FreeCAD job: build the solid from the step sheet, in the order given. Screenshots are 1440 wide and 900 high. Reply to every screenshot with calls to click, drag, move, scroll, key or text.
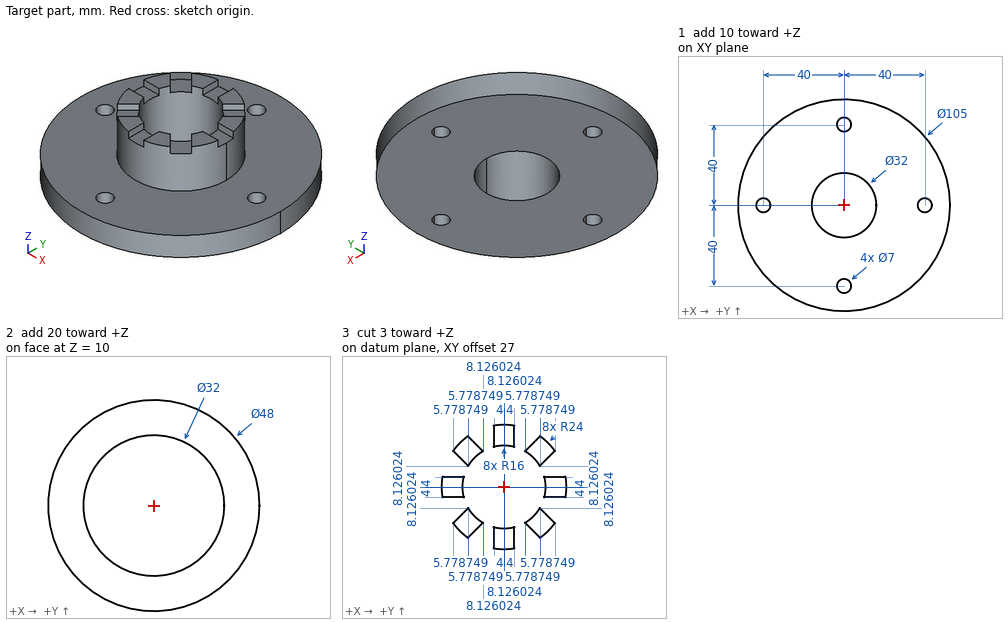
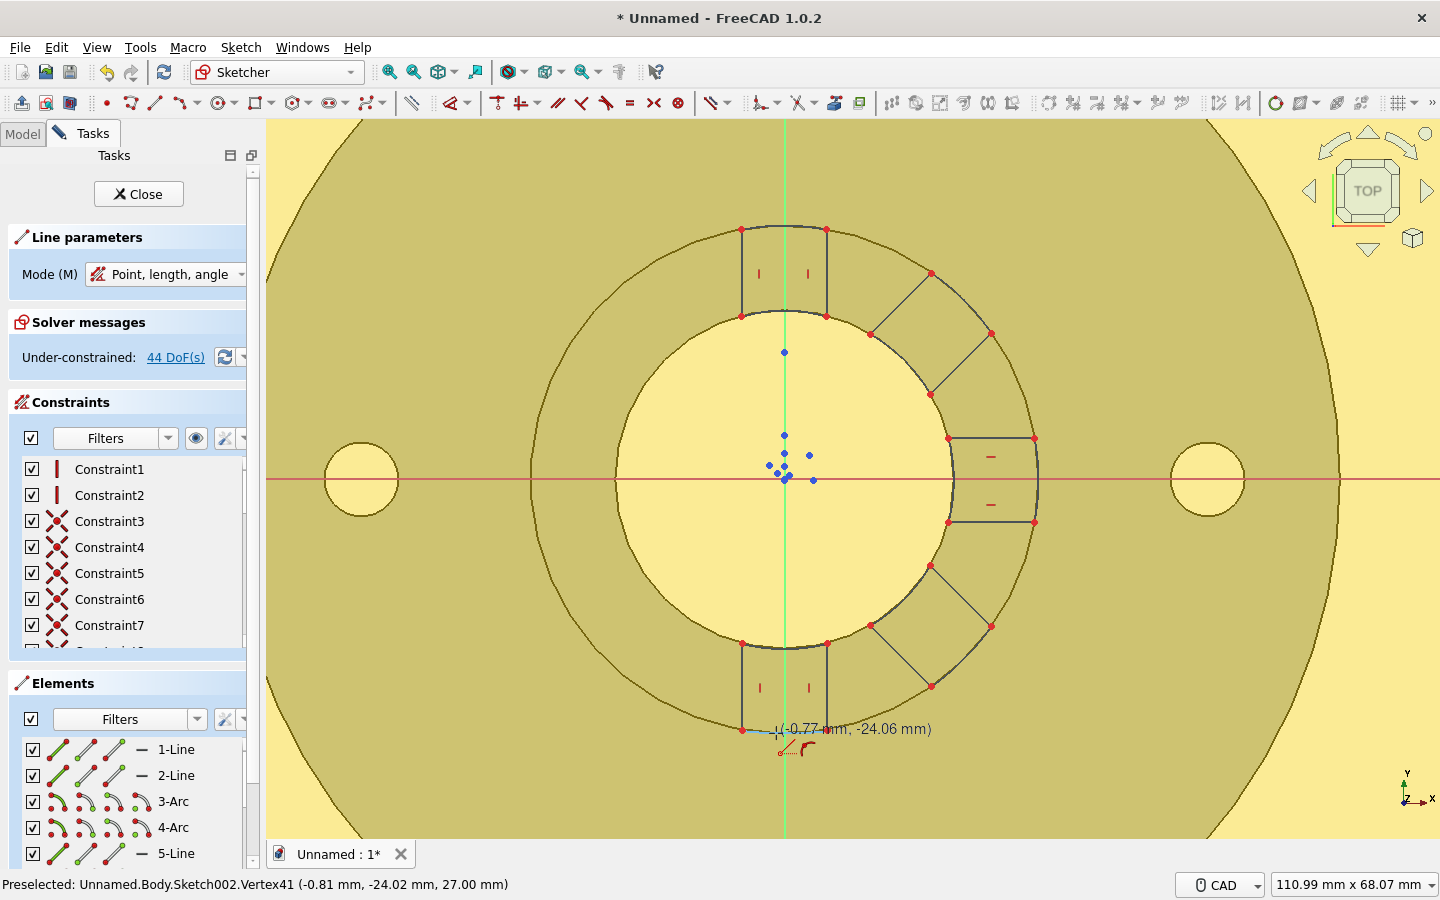
click(637, 686)
click(699, 625)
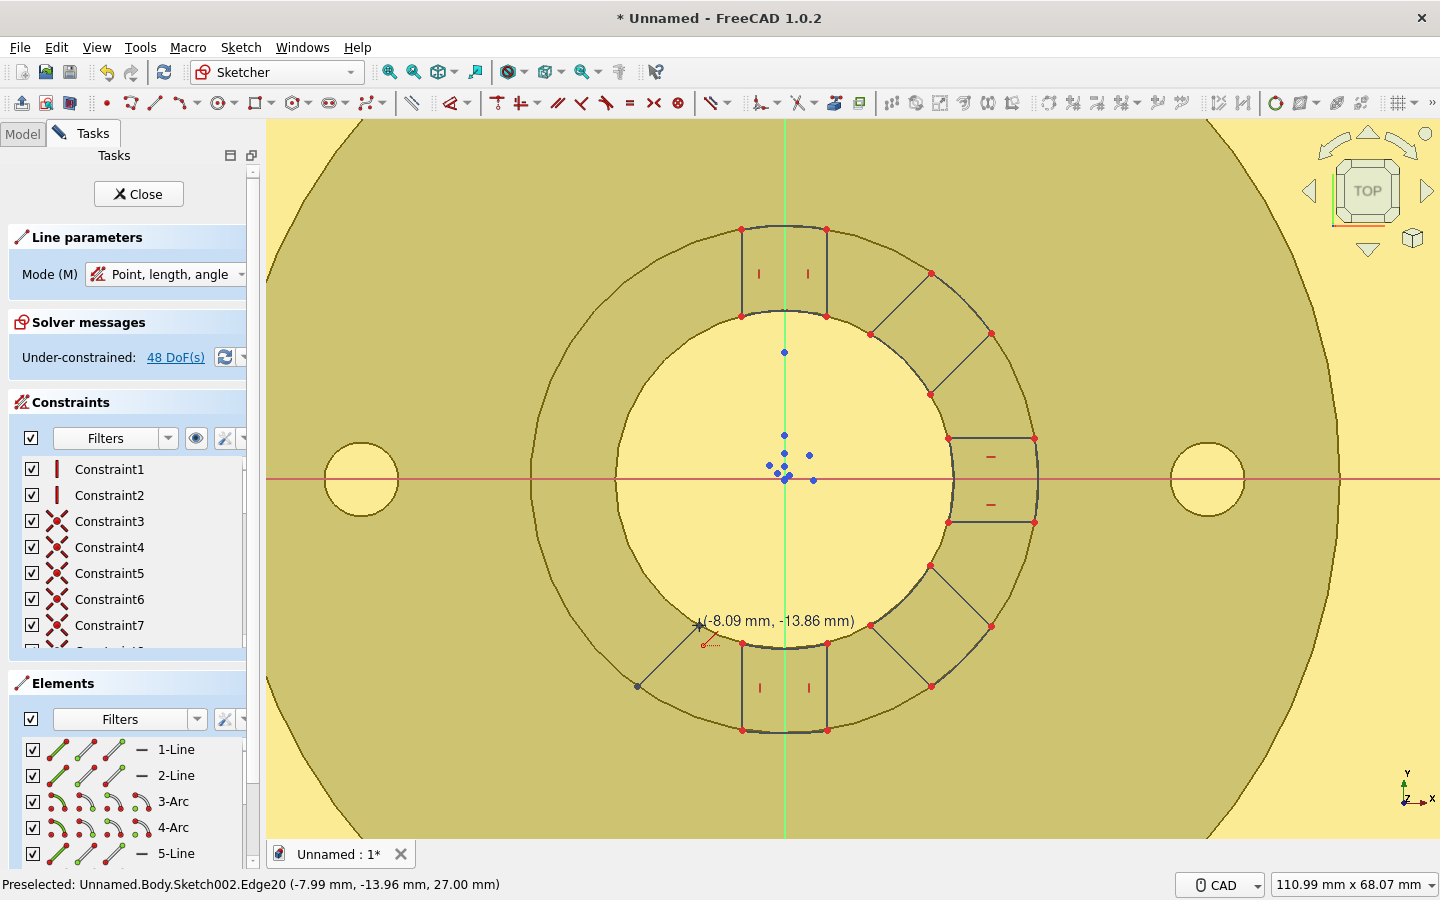
click(639, 565)
click(578, 626)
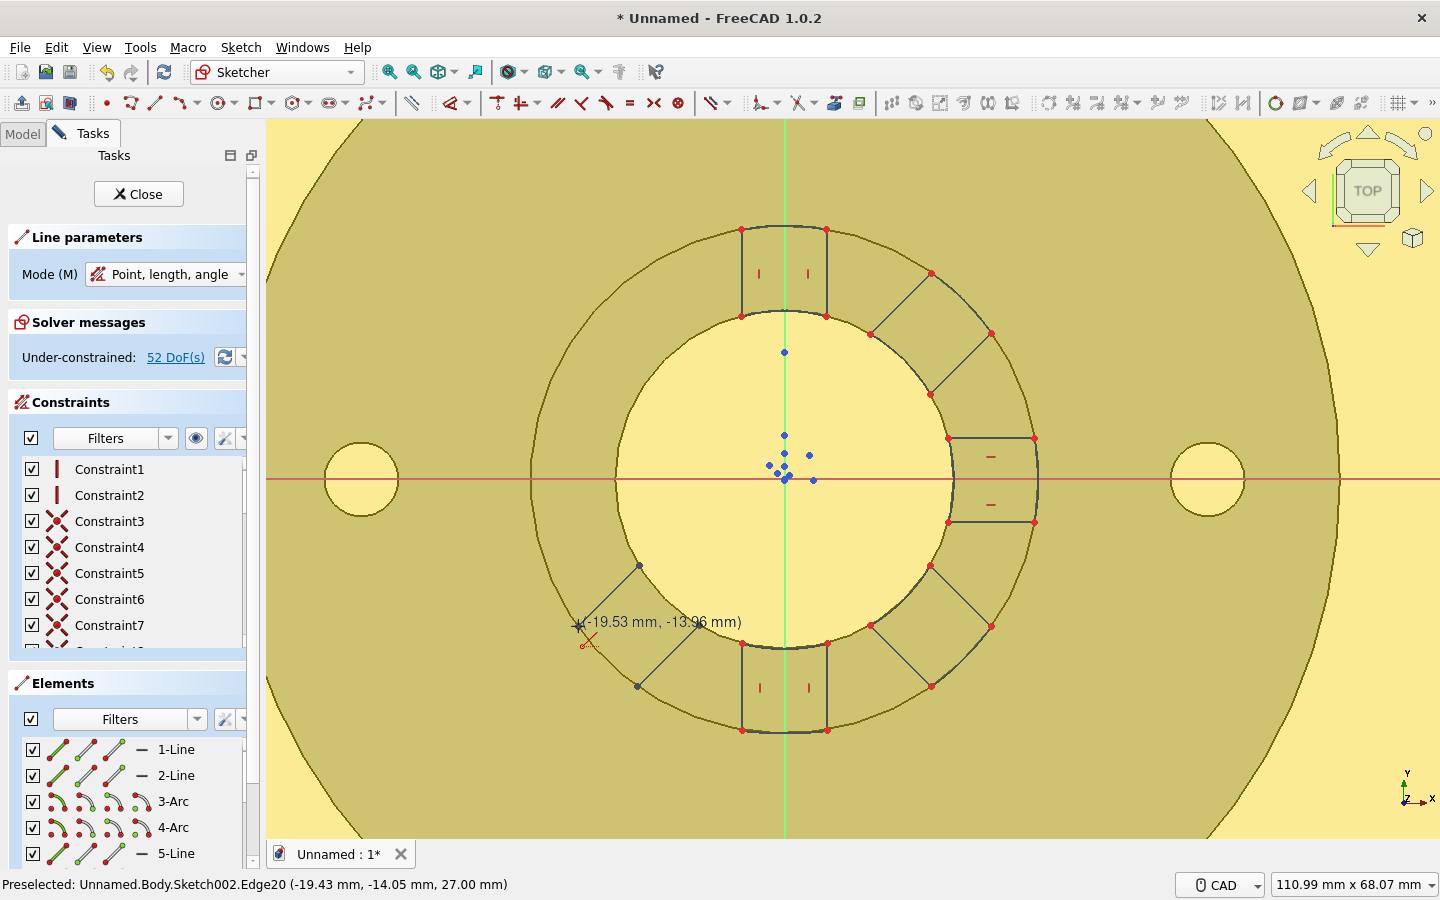
click(180, 104)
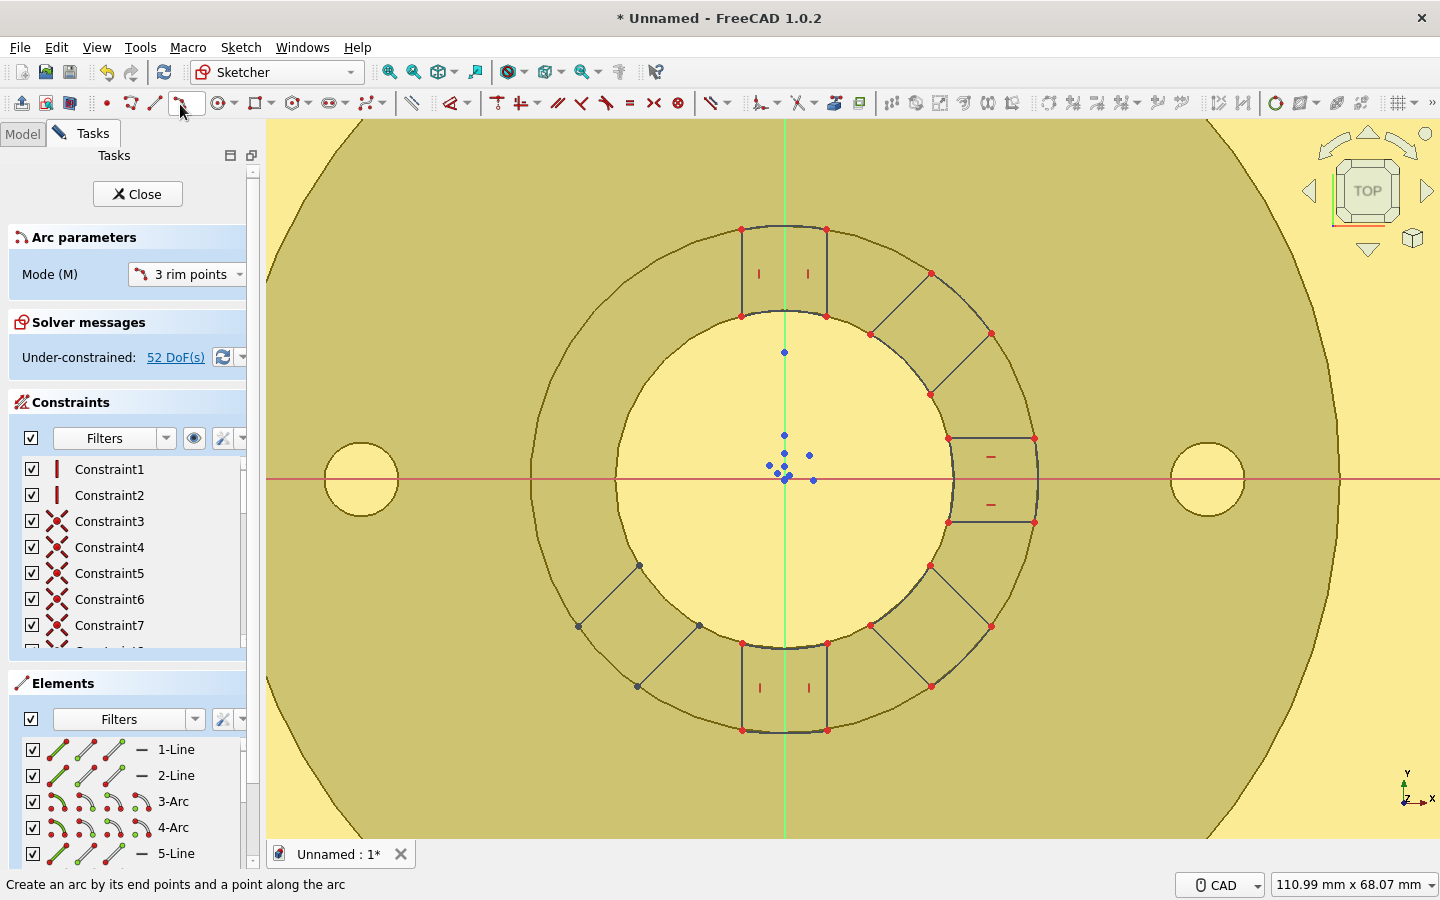
click(699, 626)
click(639, 566)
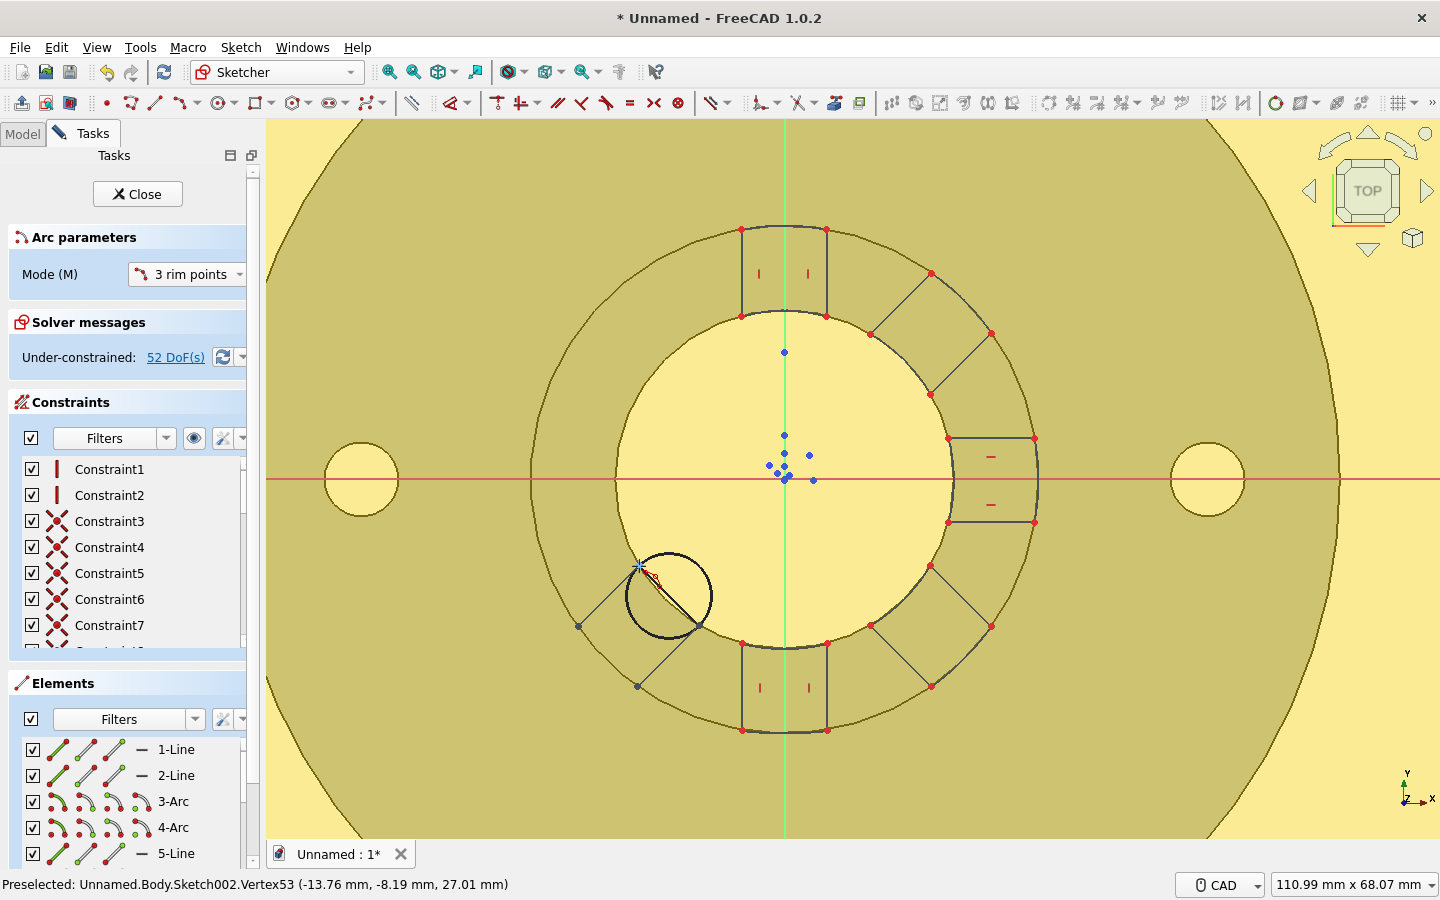
scroll(665, 599, up, 6)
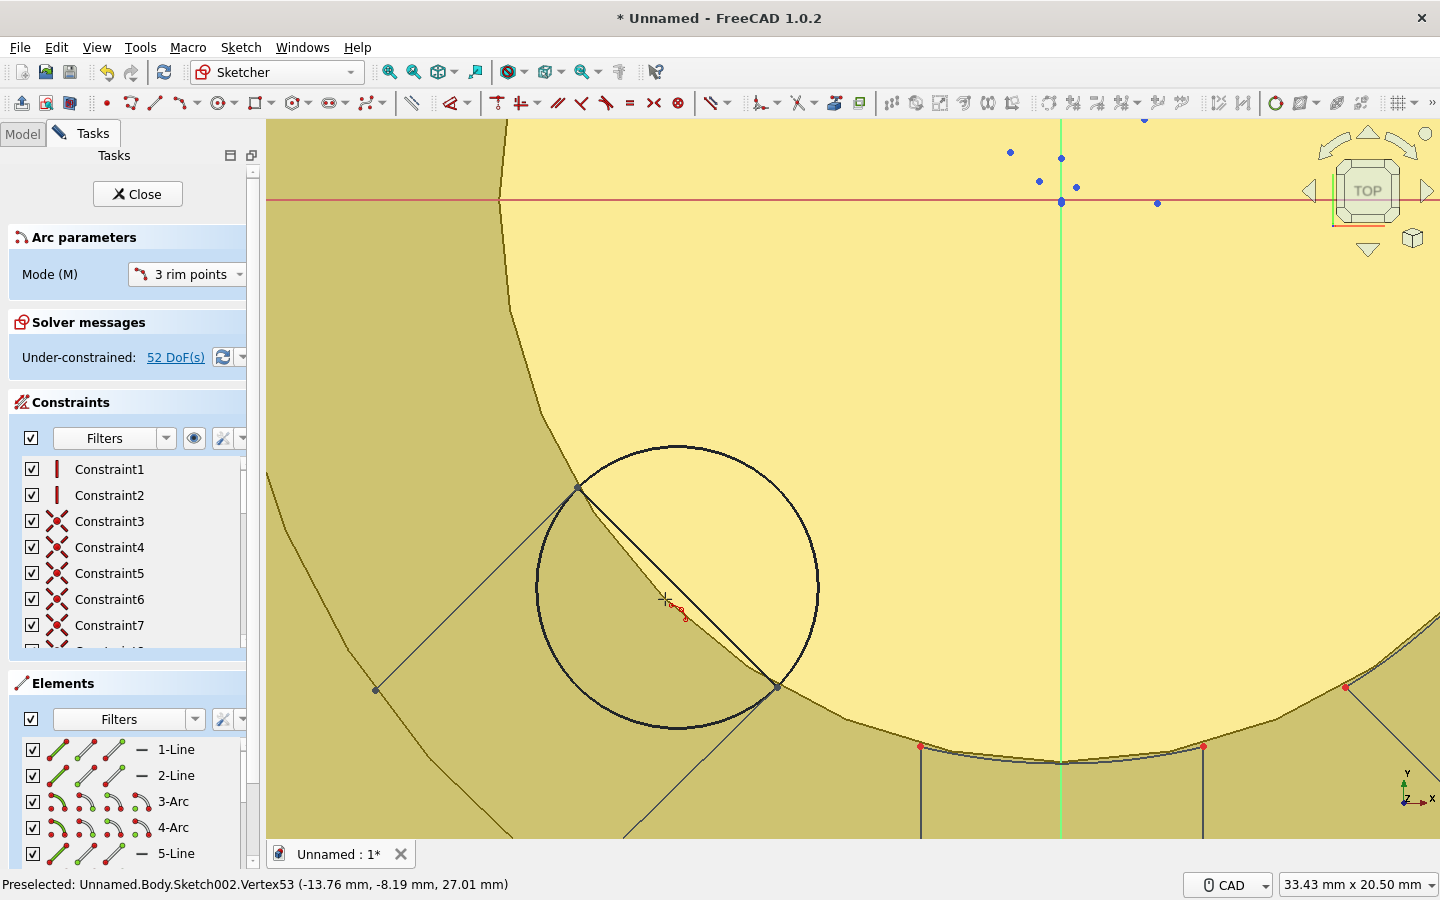
click(664, 598)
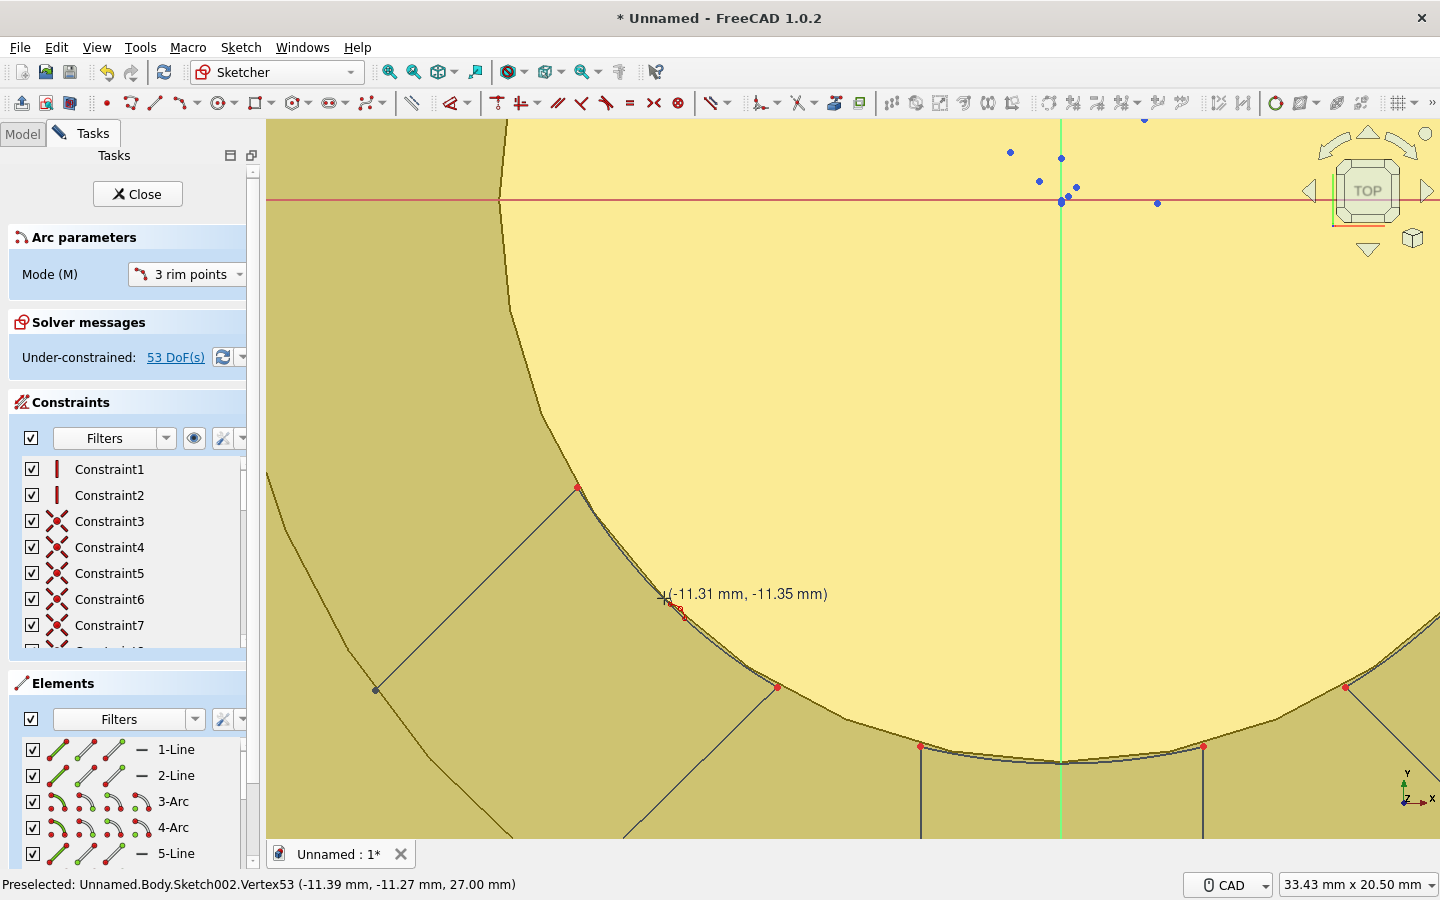
click(375, 690)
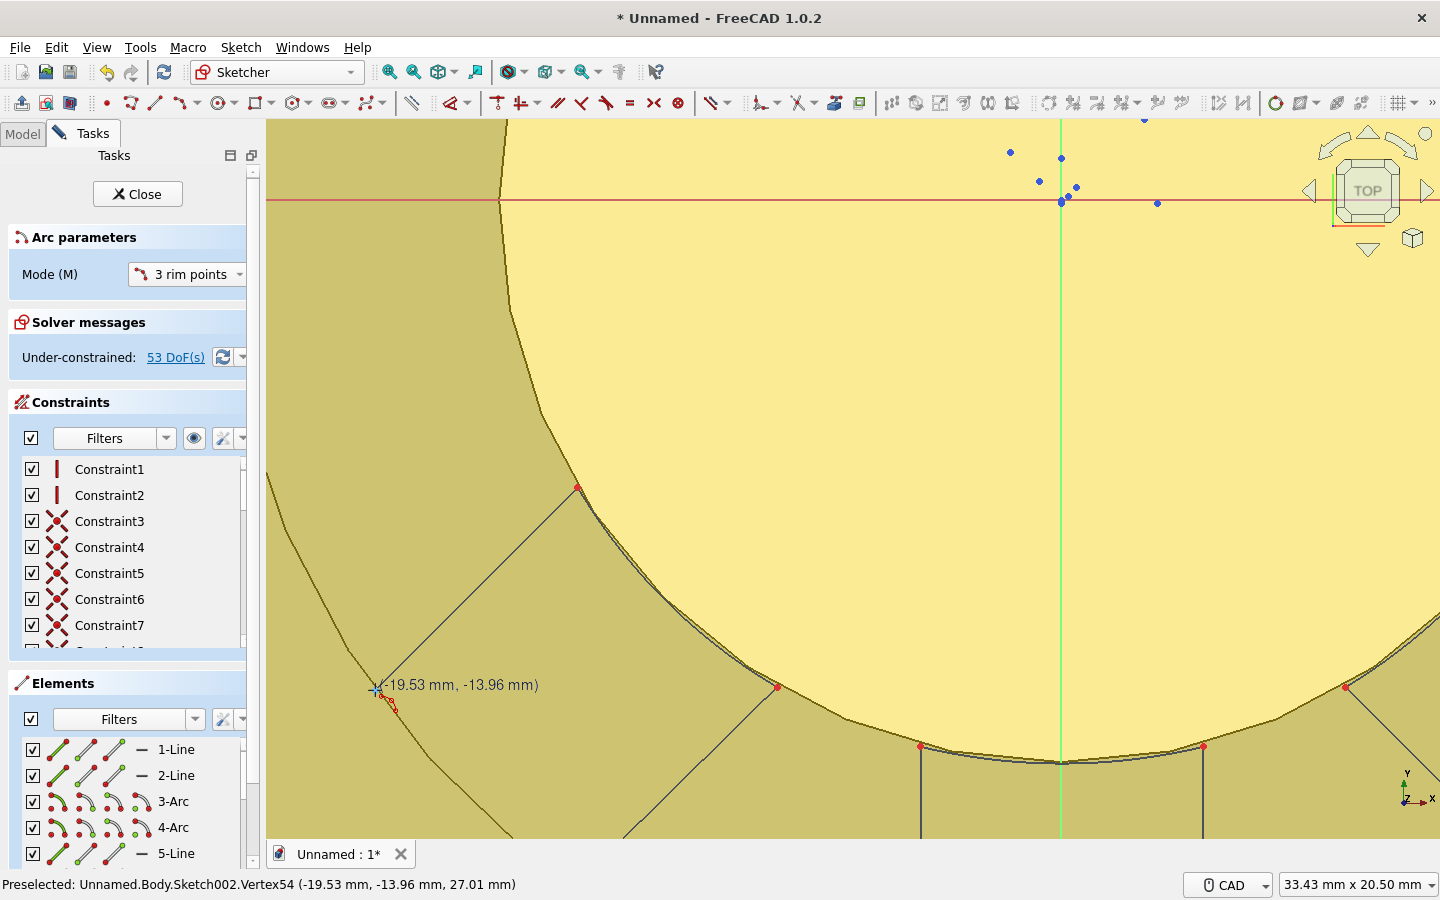
scroll(665, 599, down, 6)